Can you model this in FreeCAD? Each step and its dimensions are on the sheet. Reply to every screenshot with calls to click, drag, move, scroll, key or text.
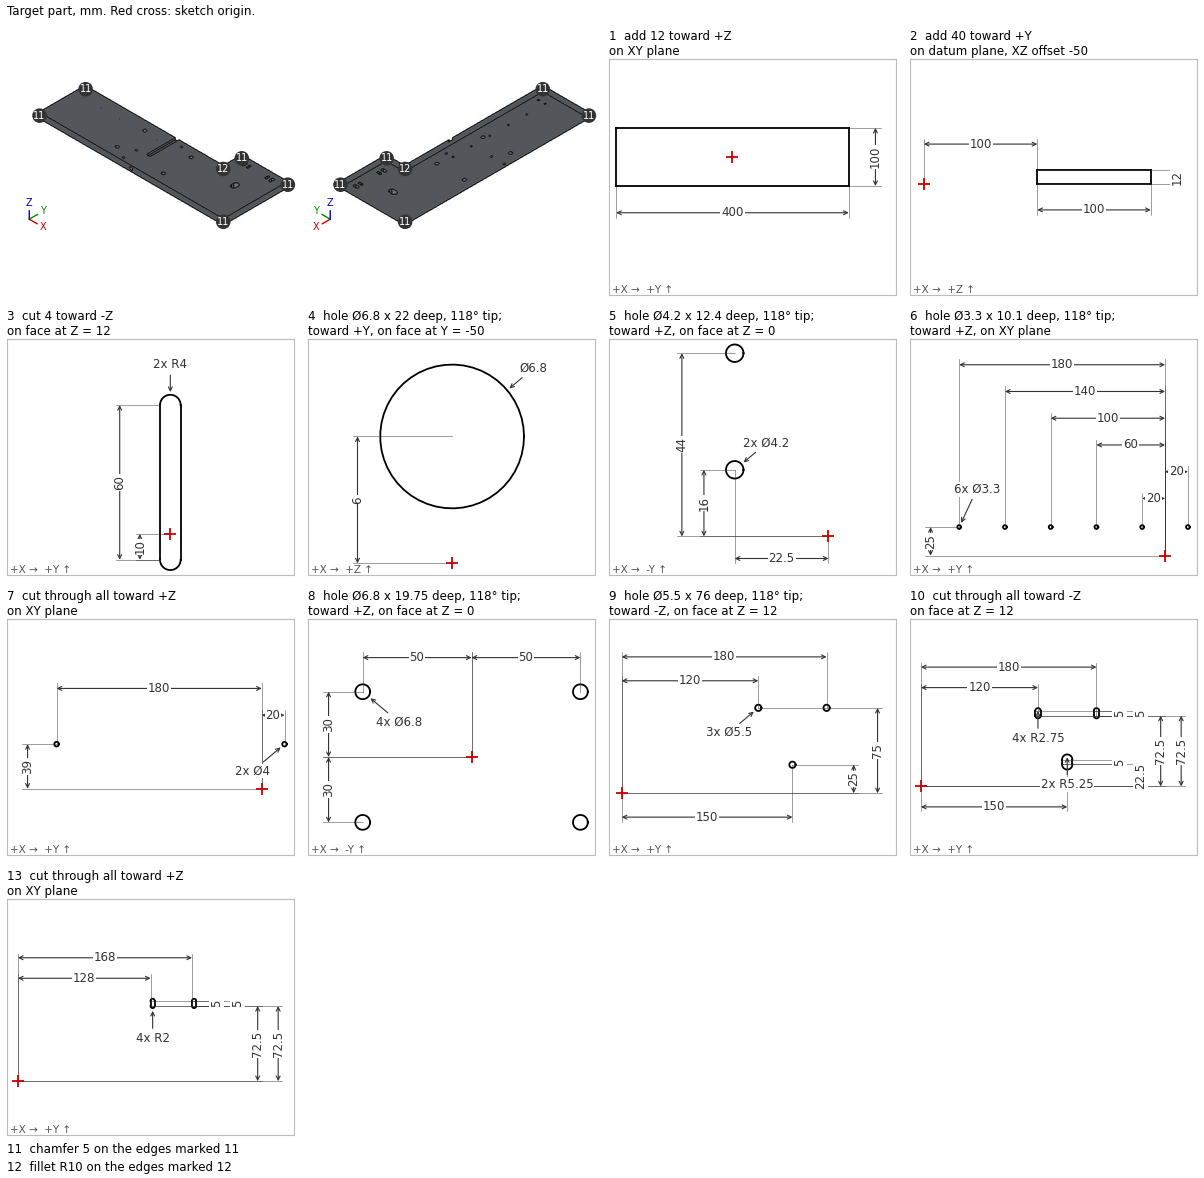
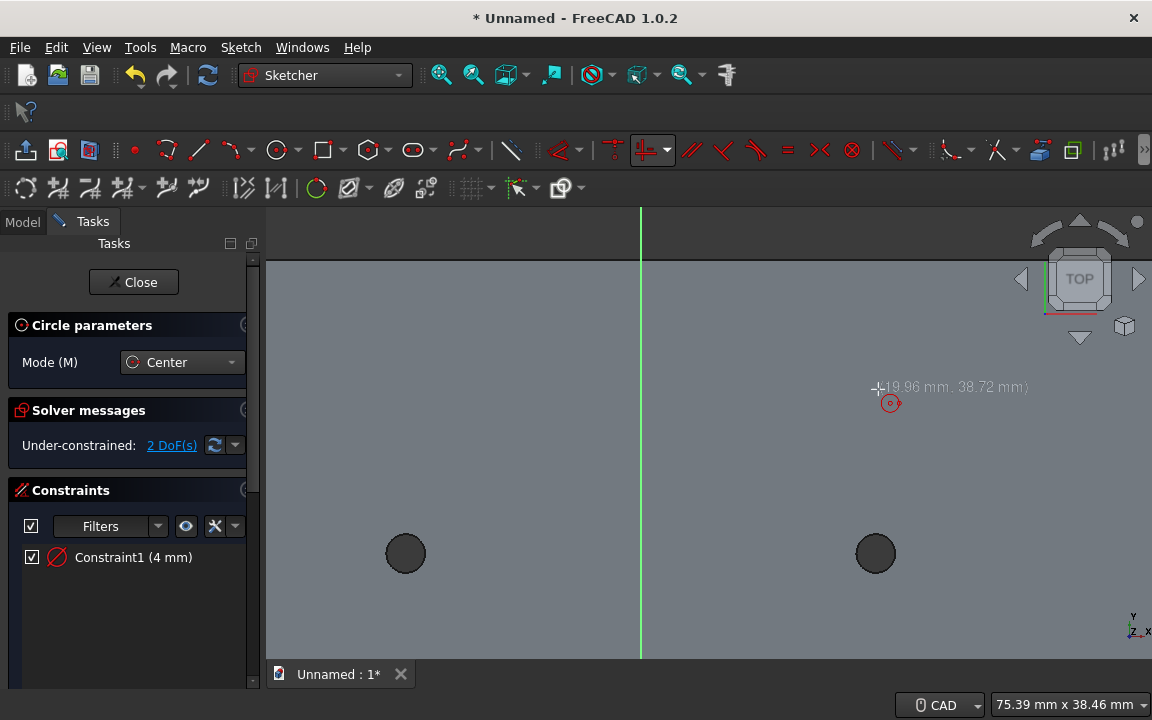
scroll(878, 389, down, 8)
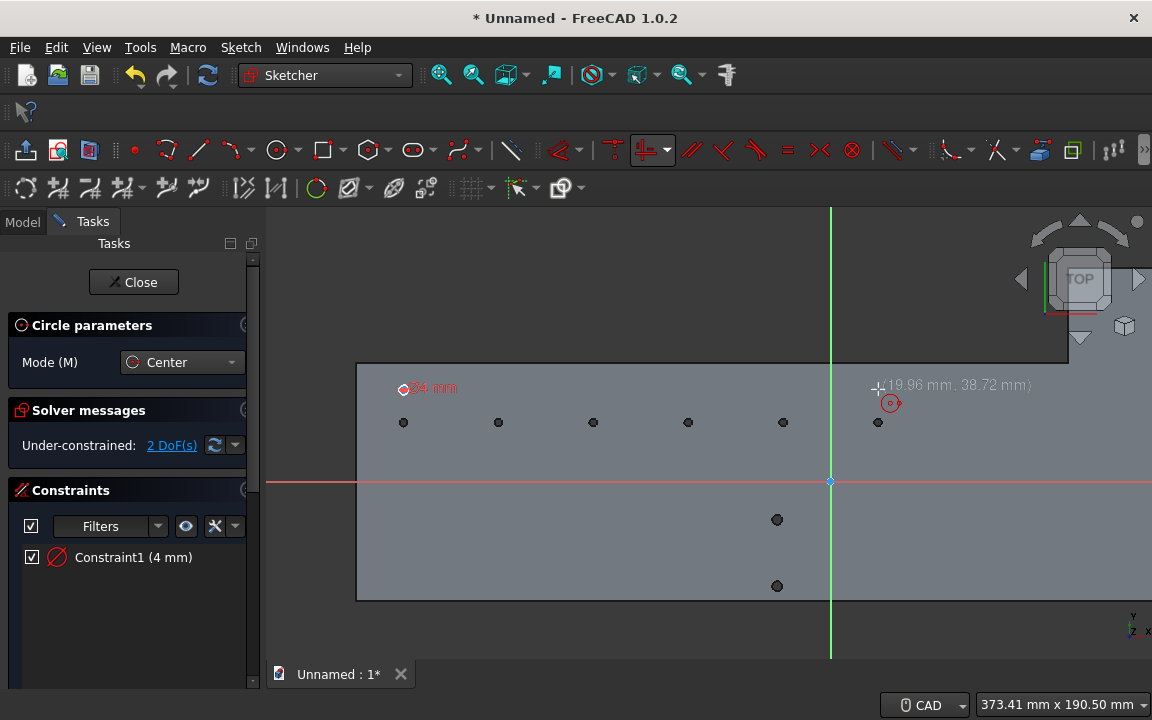
click(878, 389)
move(881, 386)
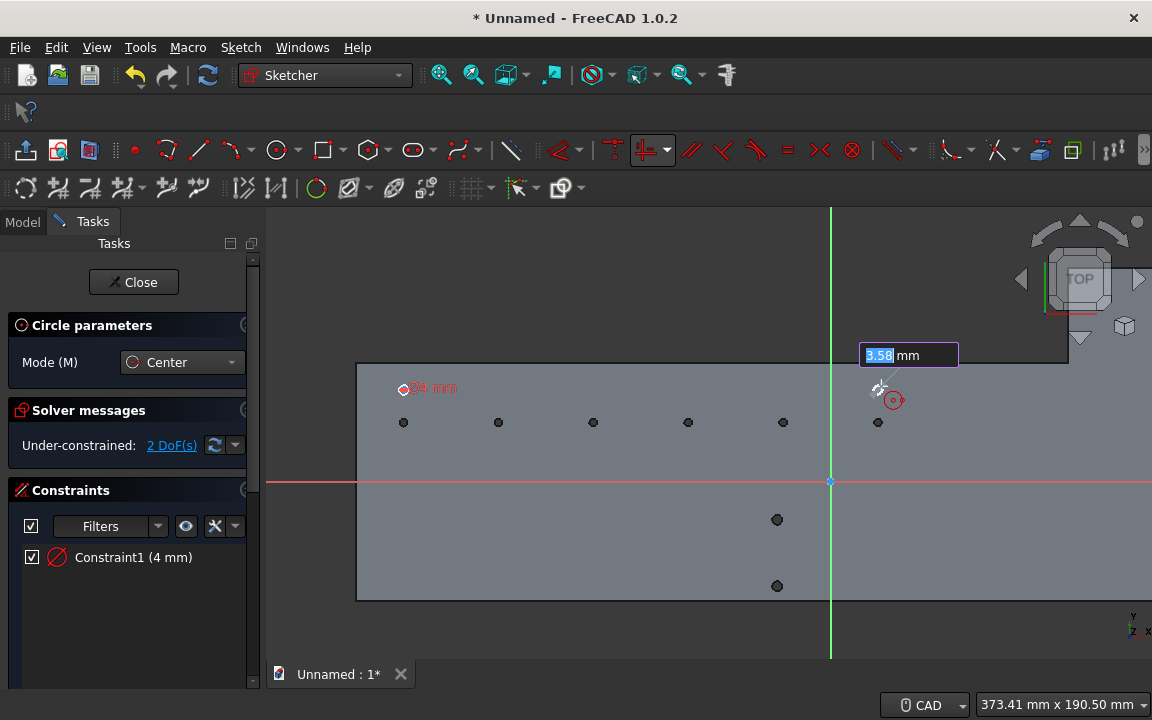
text(4)
key(Return)
key(Escape)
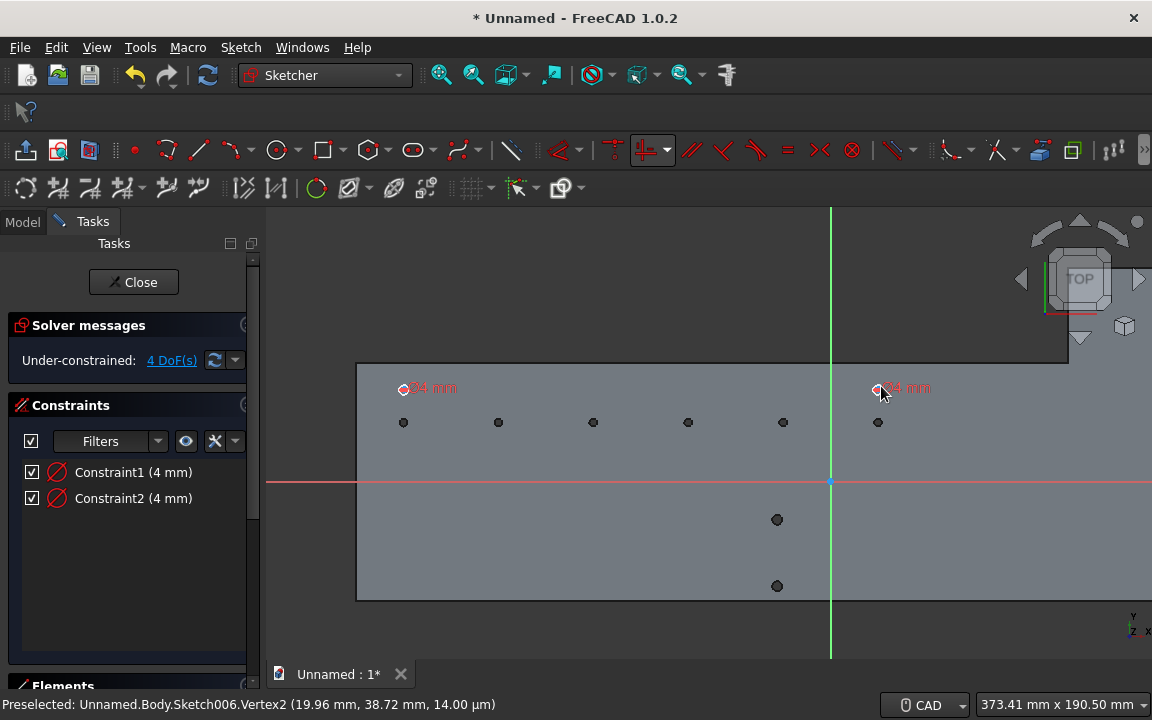
click(404, 390)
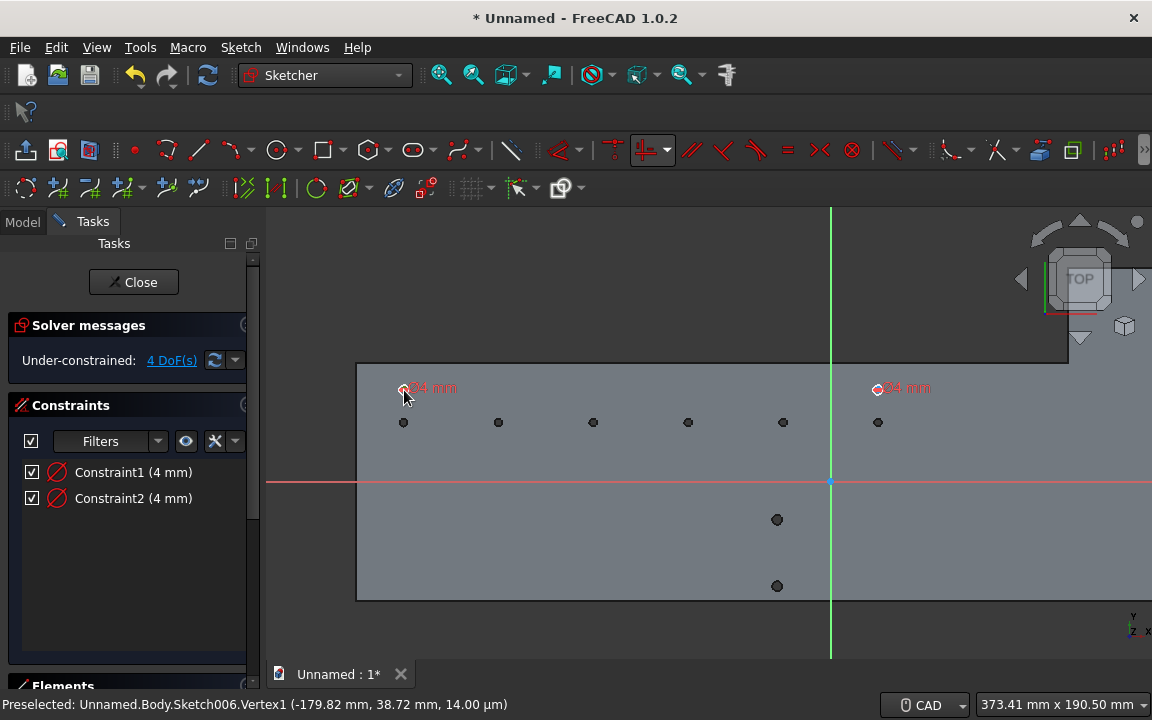
click(878, 390)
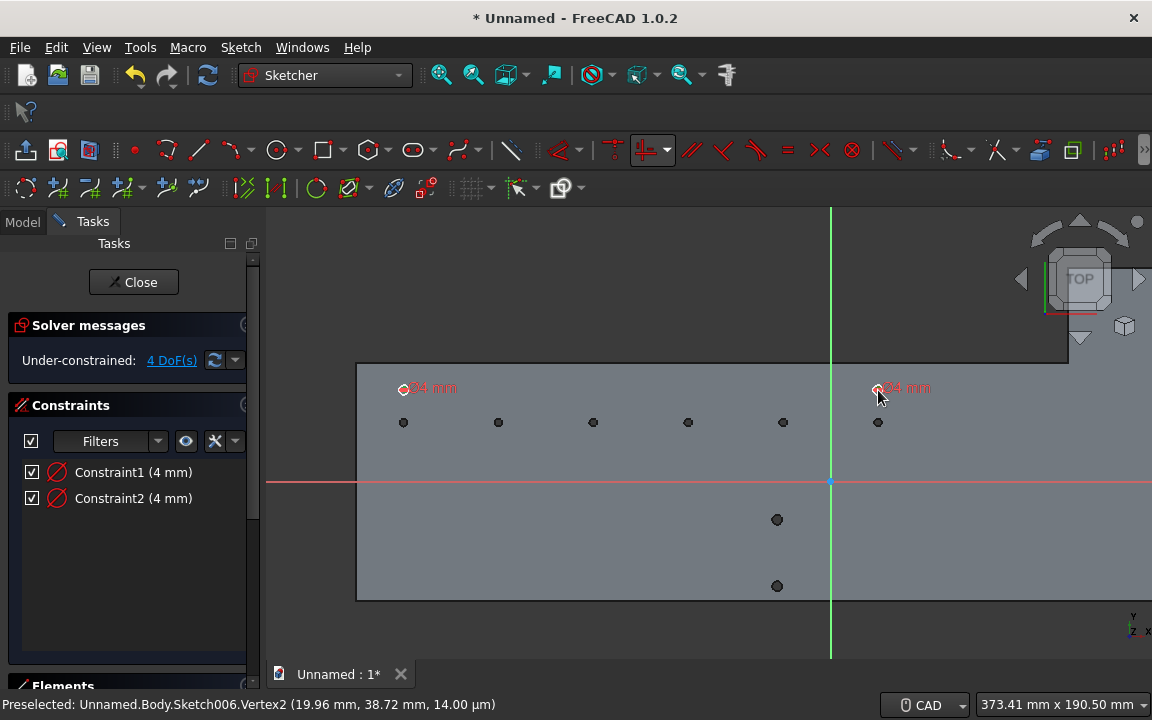
click(670, 150)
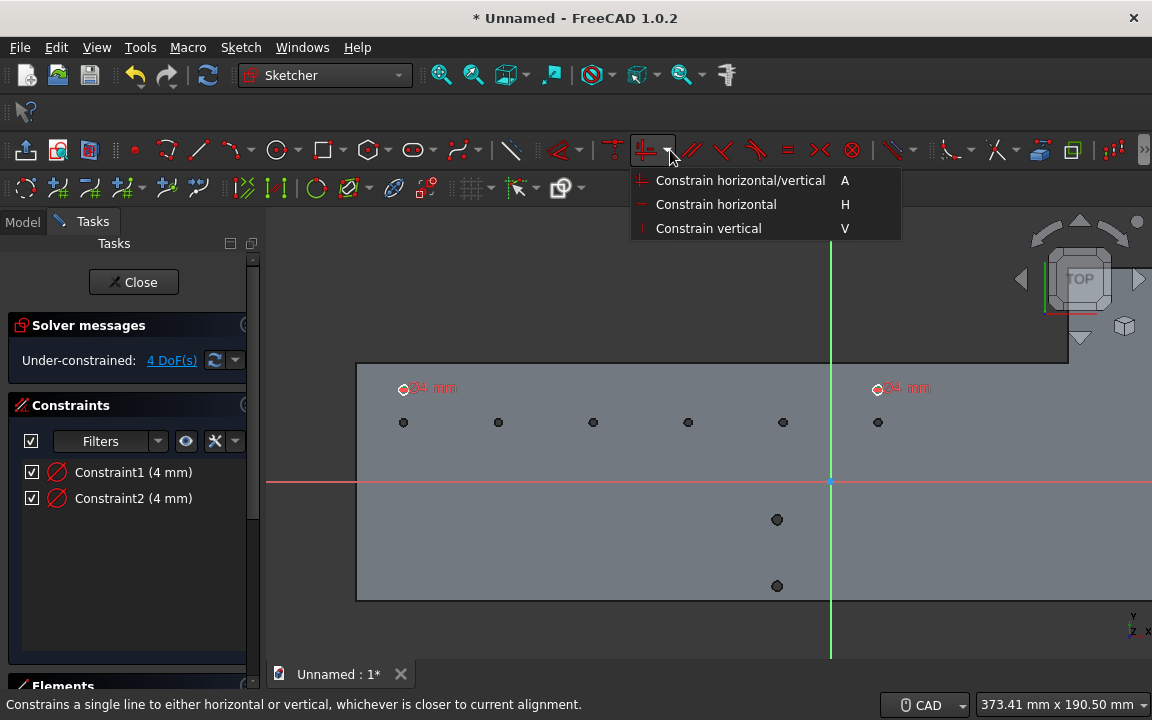
click(766, 204)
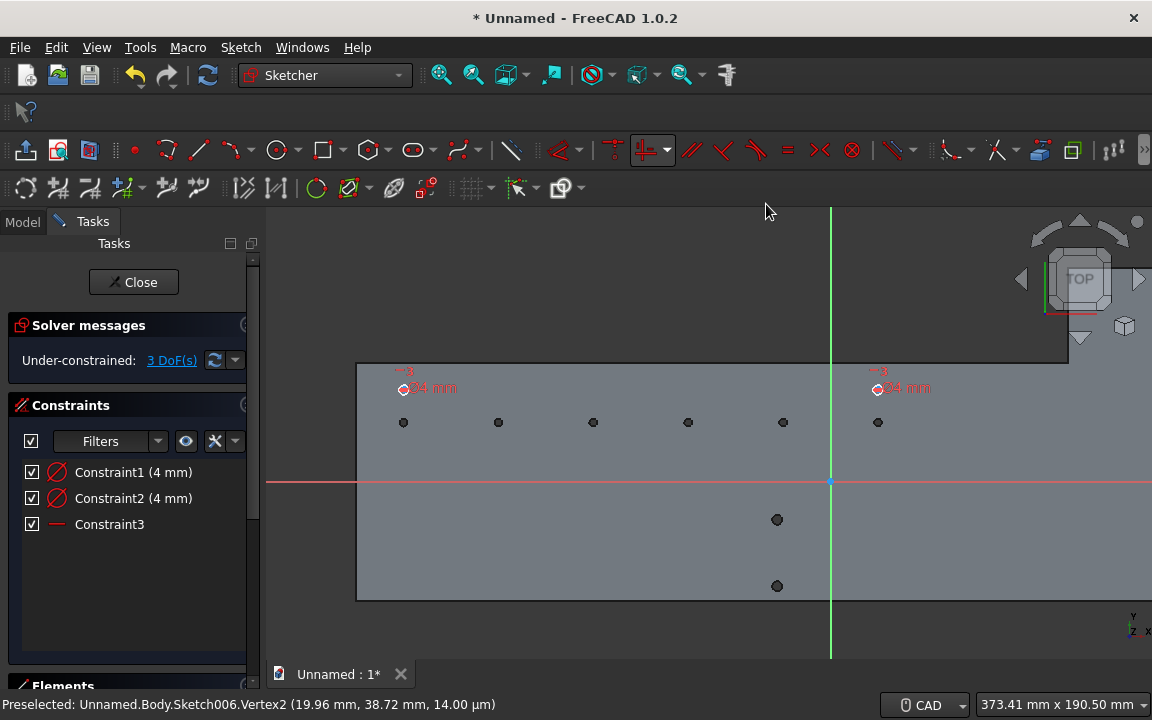
click(558, 150)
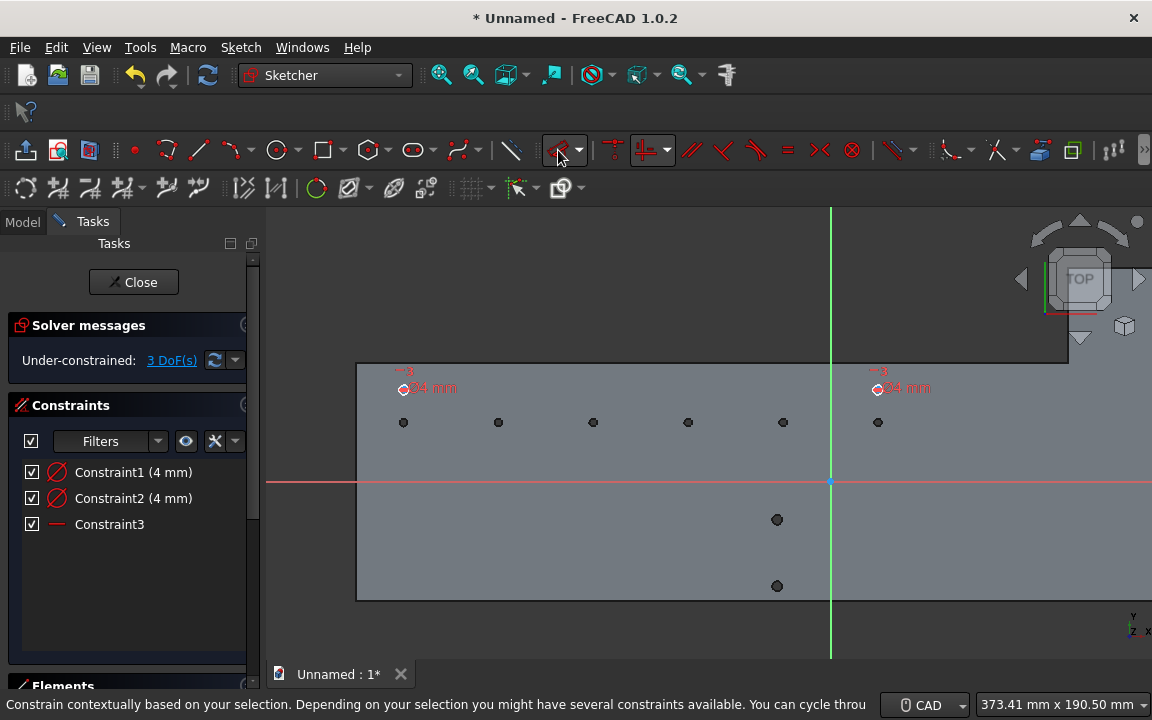
click(404, 390)
click(370, 436)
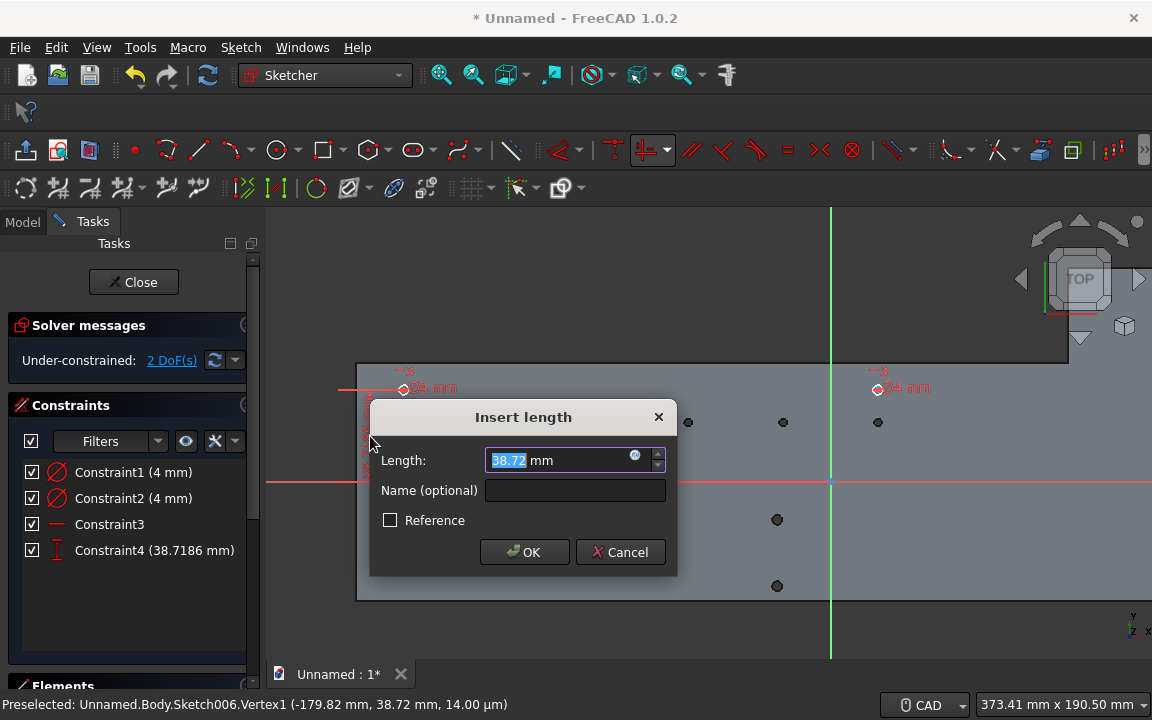
text(39)
key(Return)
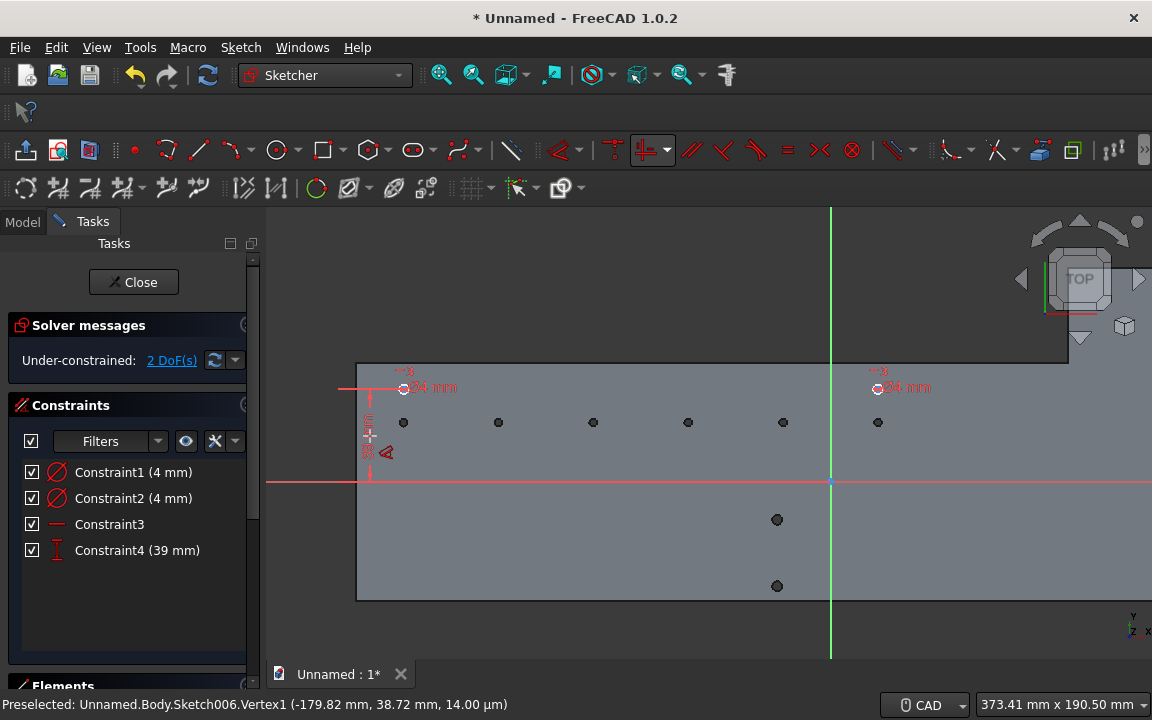
click(878, 389)
click(854, 516)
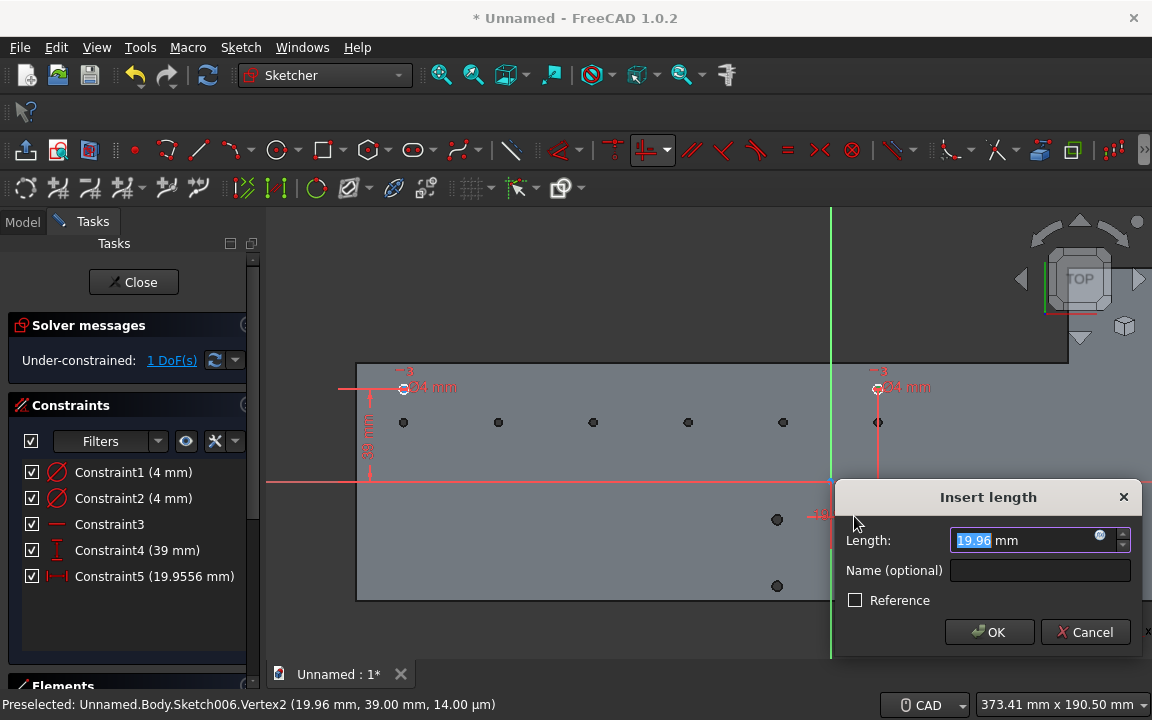
text(20)
key(Return)